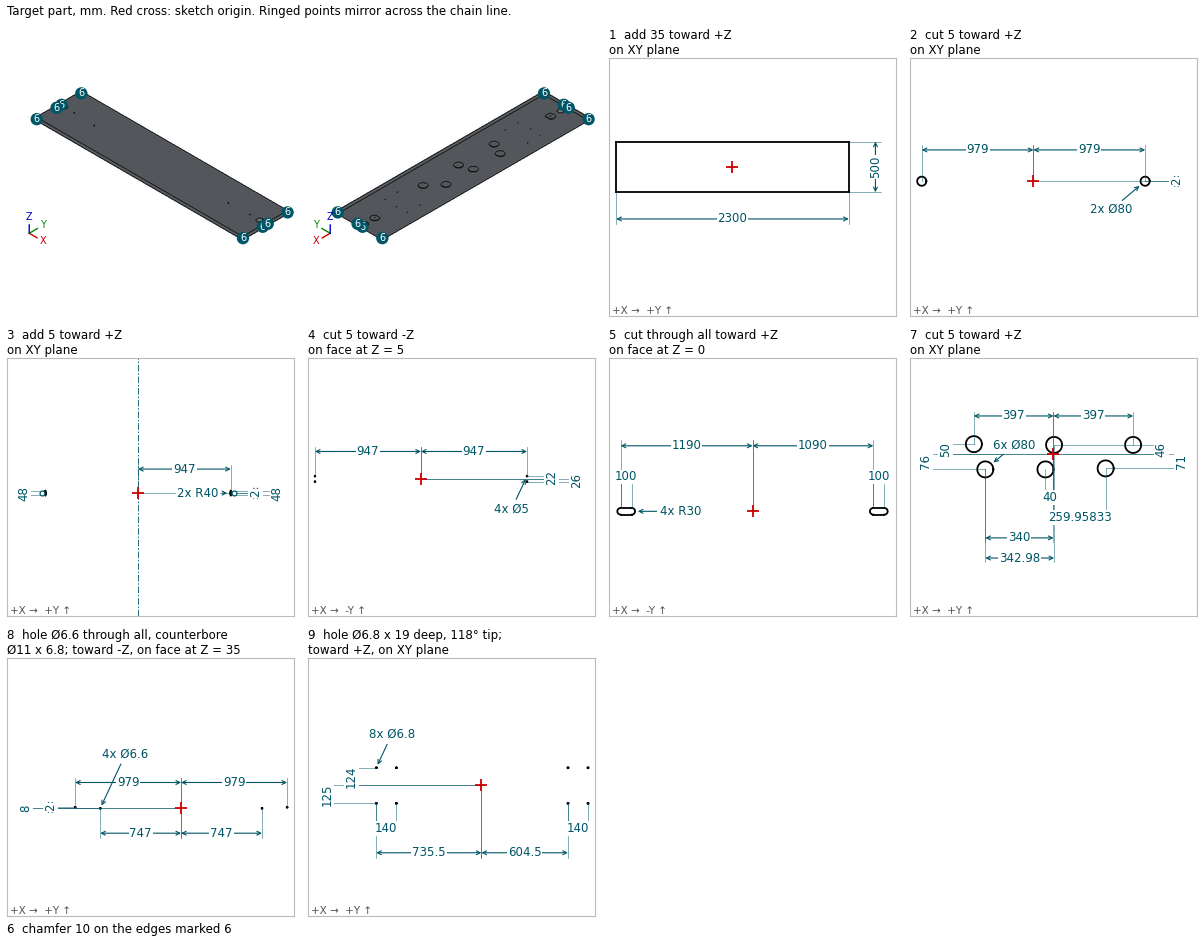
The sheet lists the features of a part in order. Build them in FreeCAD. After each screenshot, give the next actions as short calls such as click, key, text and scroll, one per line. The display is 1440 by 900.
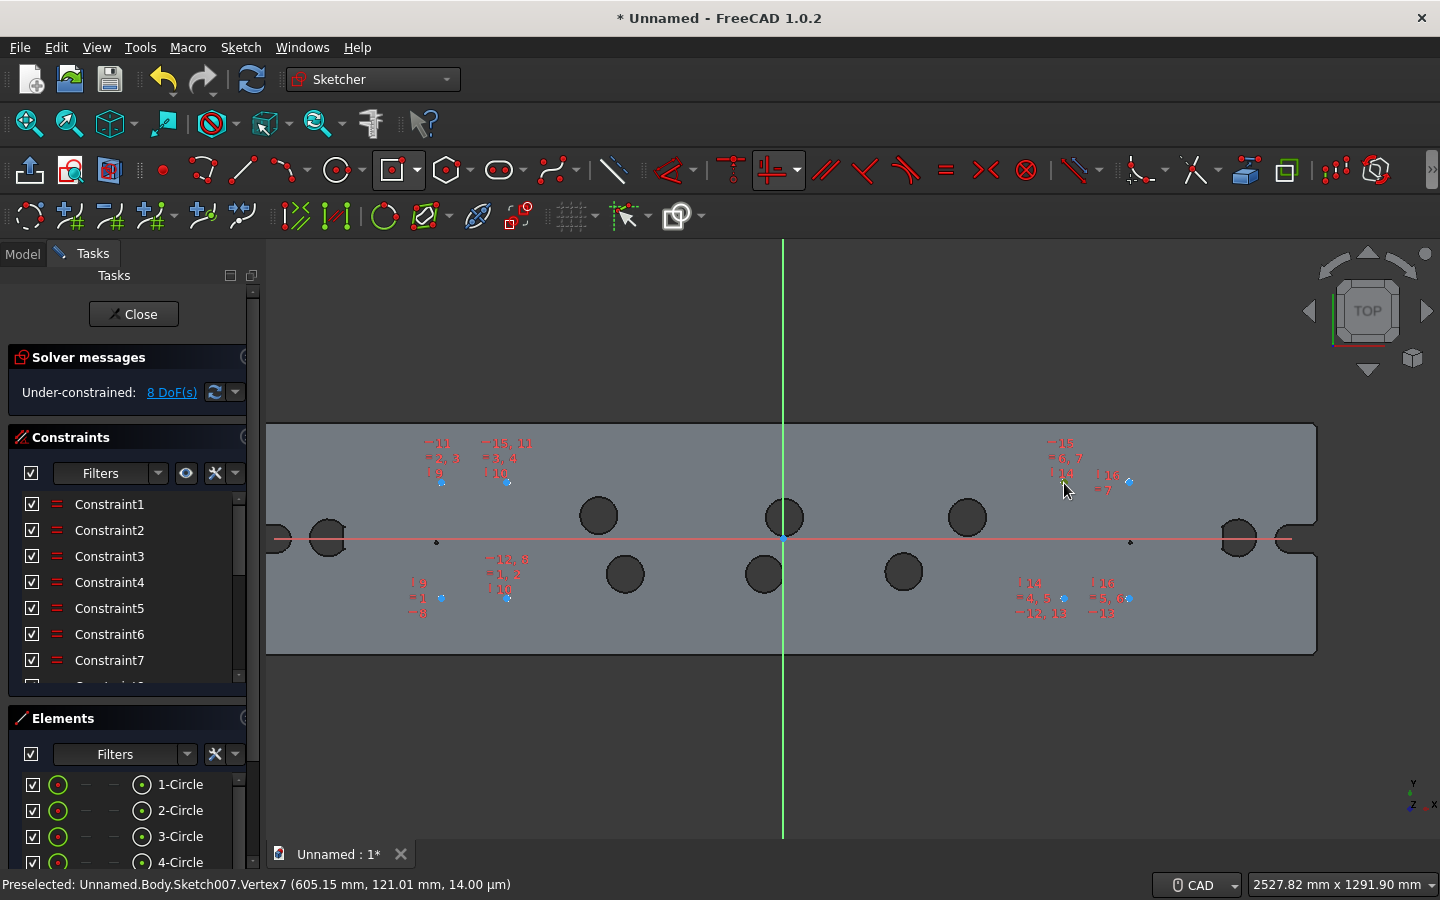
click(1129, 482)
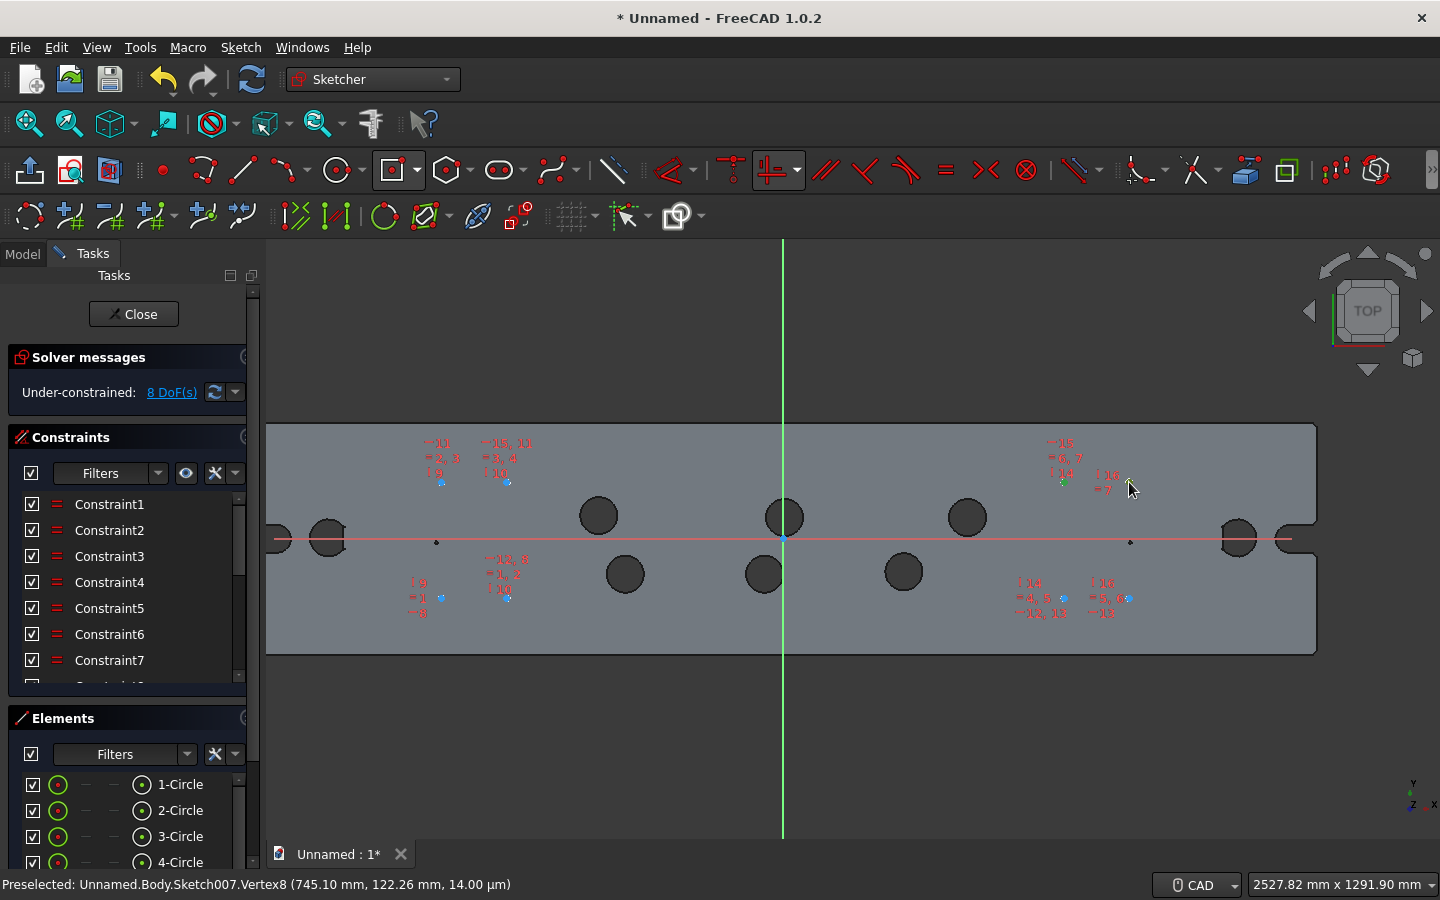
click(800, 170)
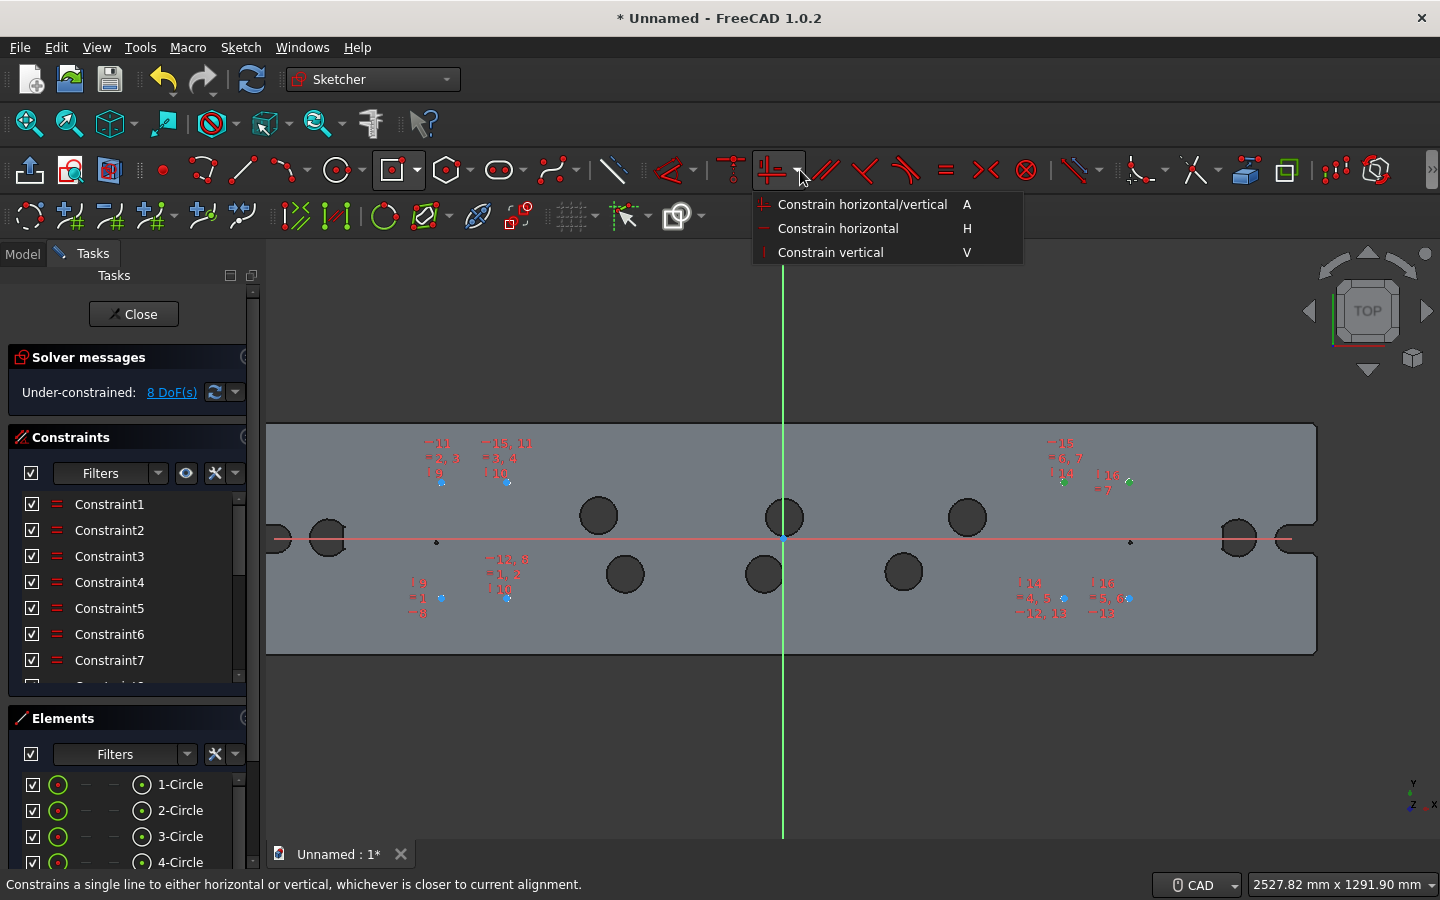
click(888, 228)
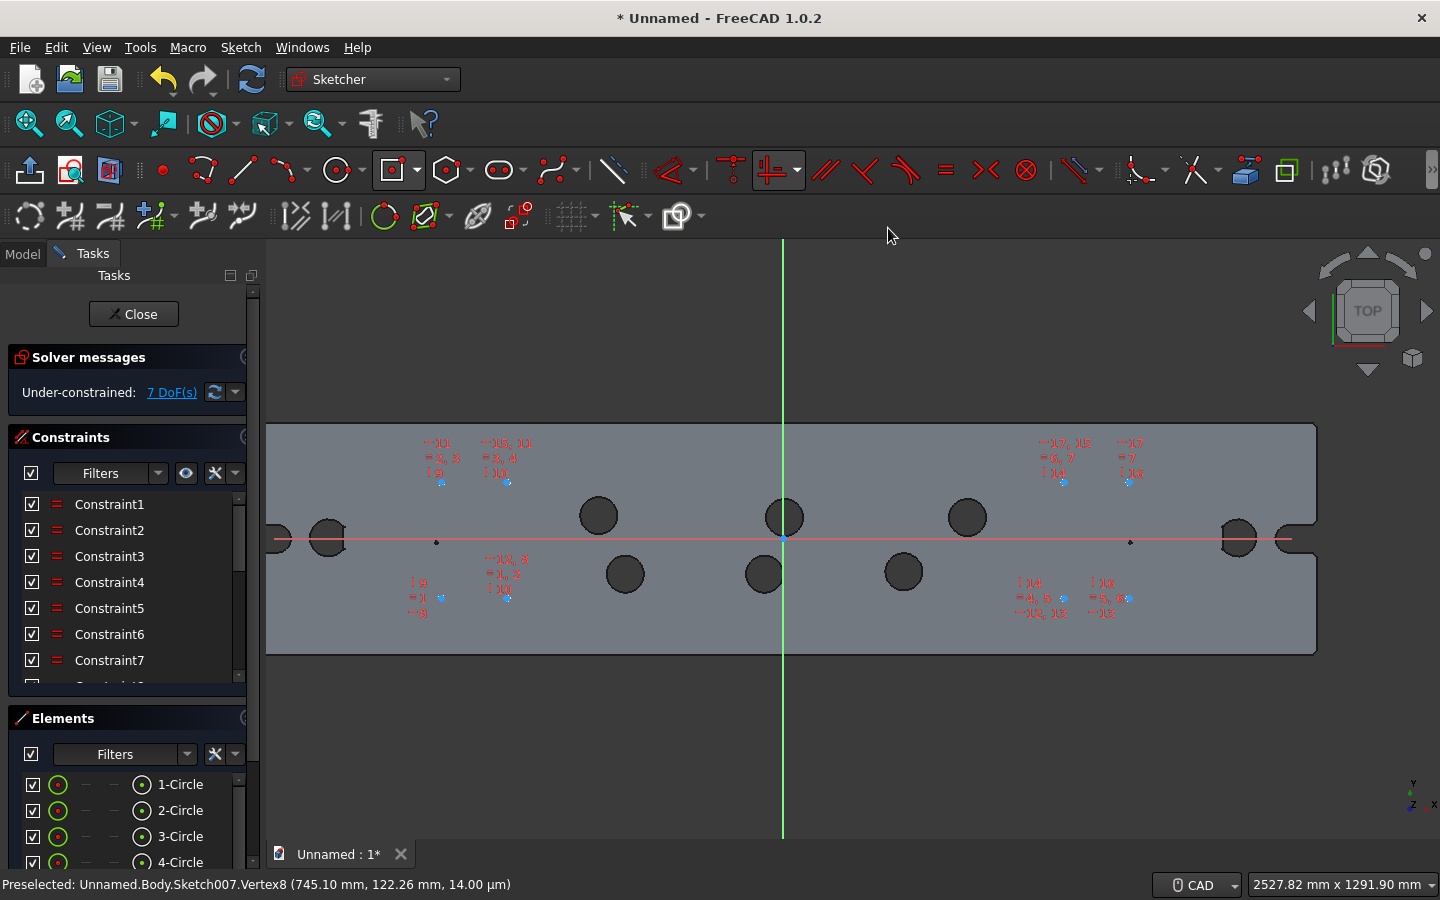
click(668, 170)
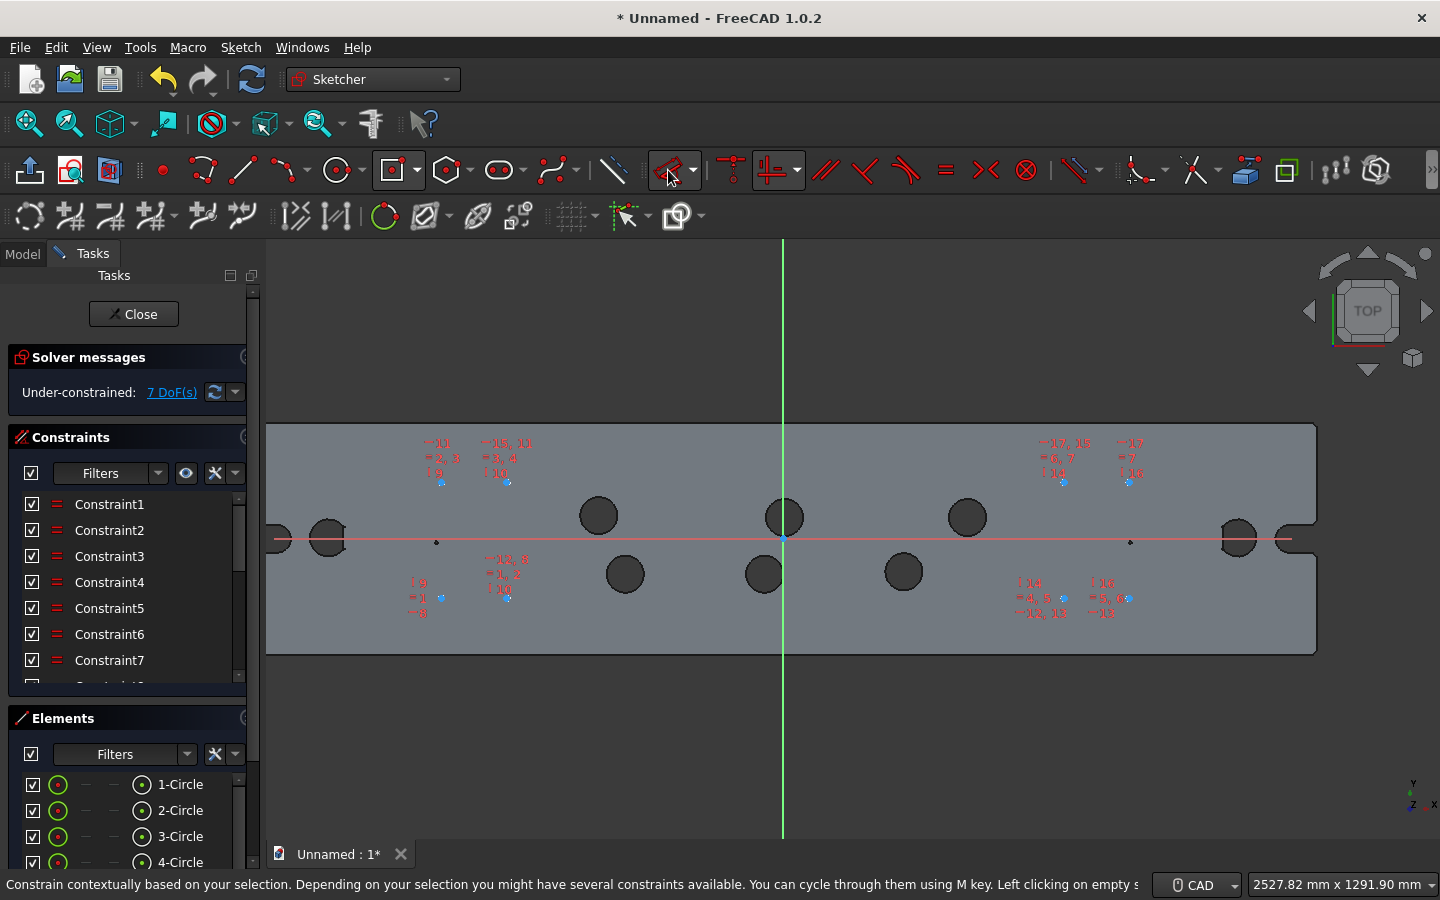
scroll(439, 600, up, 13)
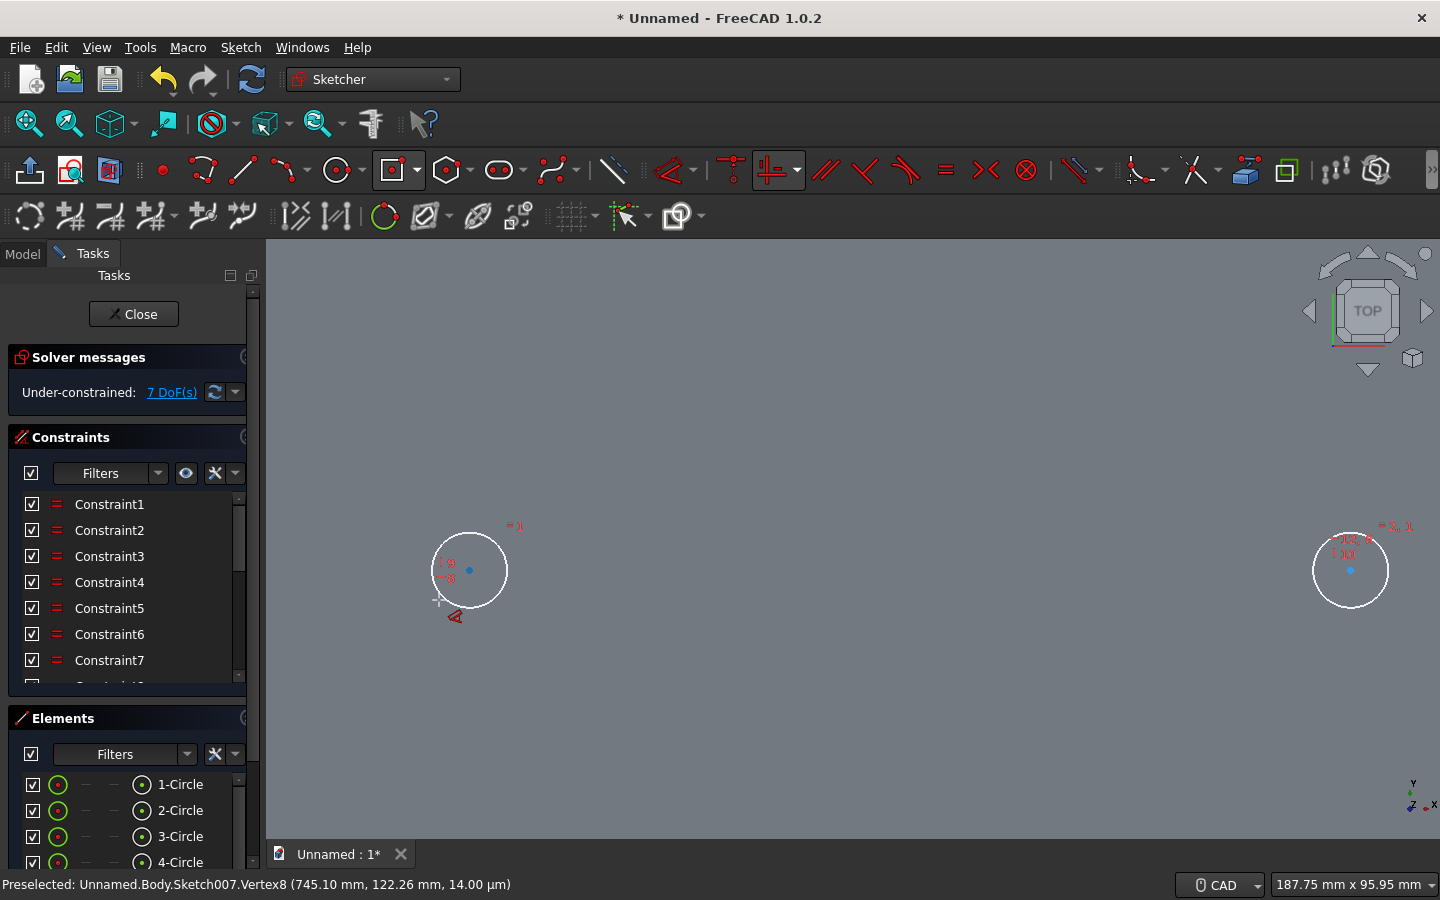
click(443, 597)
click(420, 620)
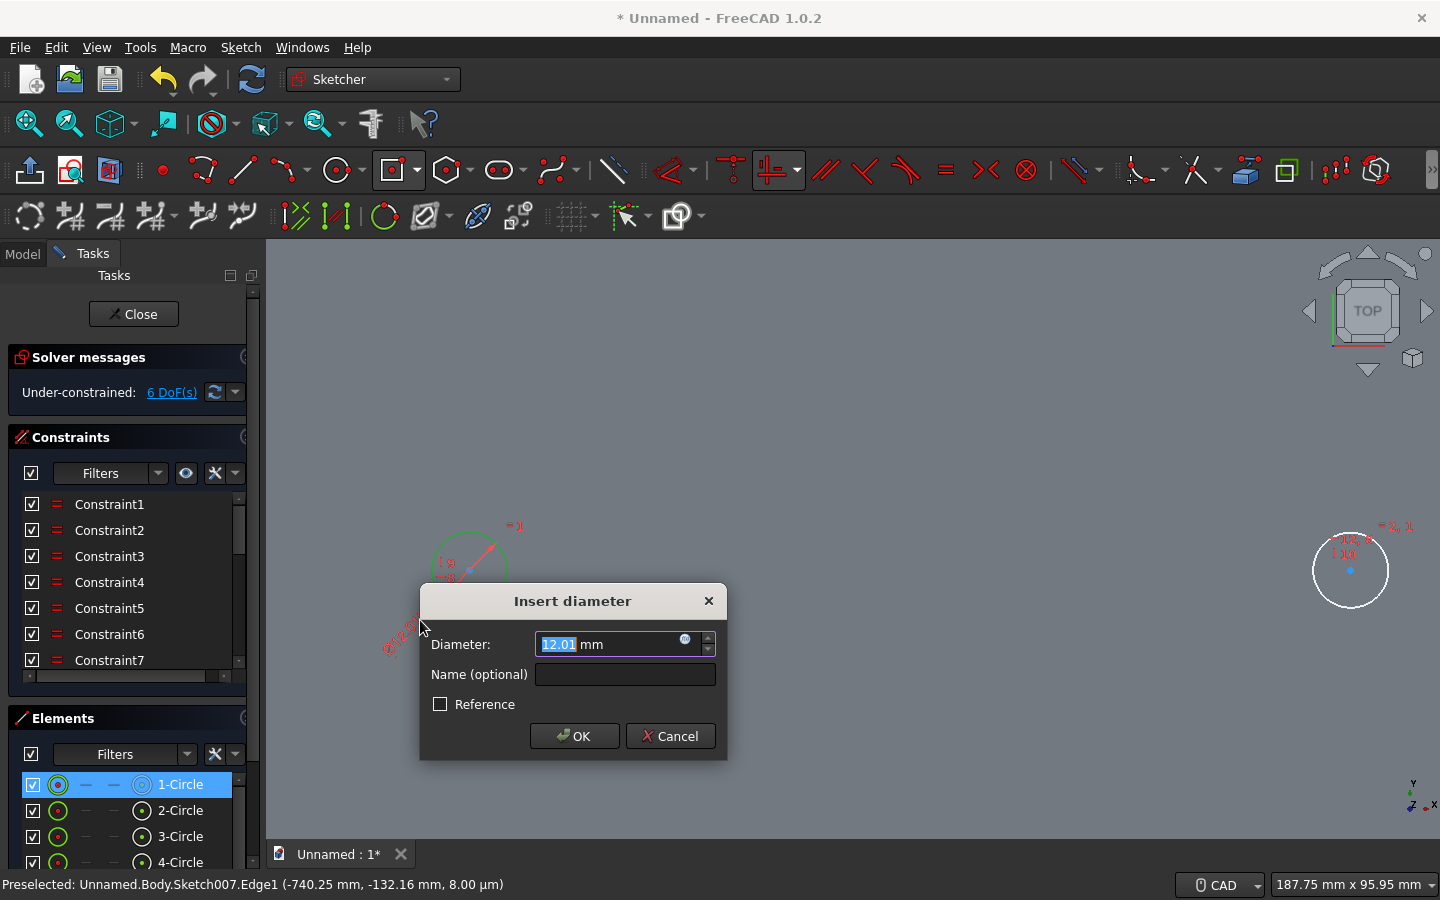
text(6.8)
key(Return)